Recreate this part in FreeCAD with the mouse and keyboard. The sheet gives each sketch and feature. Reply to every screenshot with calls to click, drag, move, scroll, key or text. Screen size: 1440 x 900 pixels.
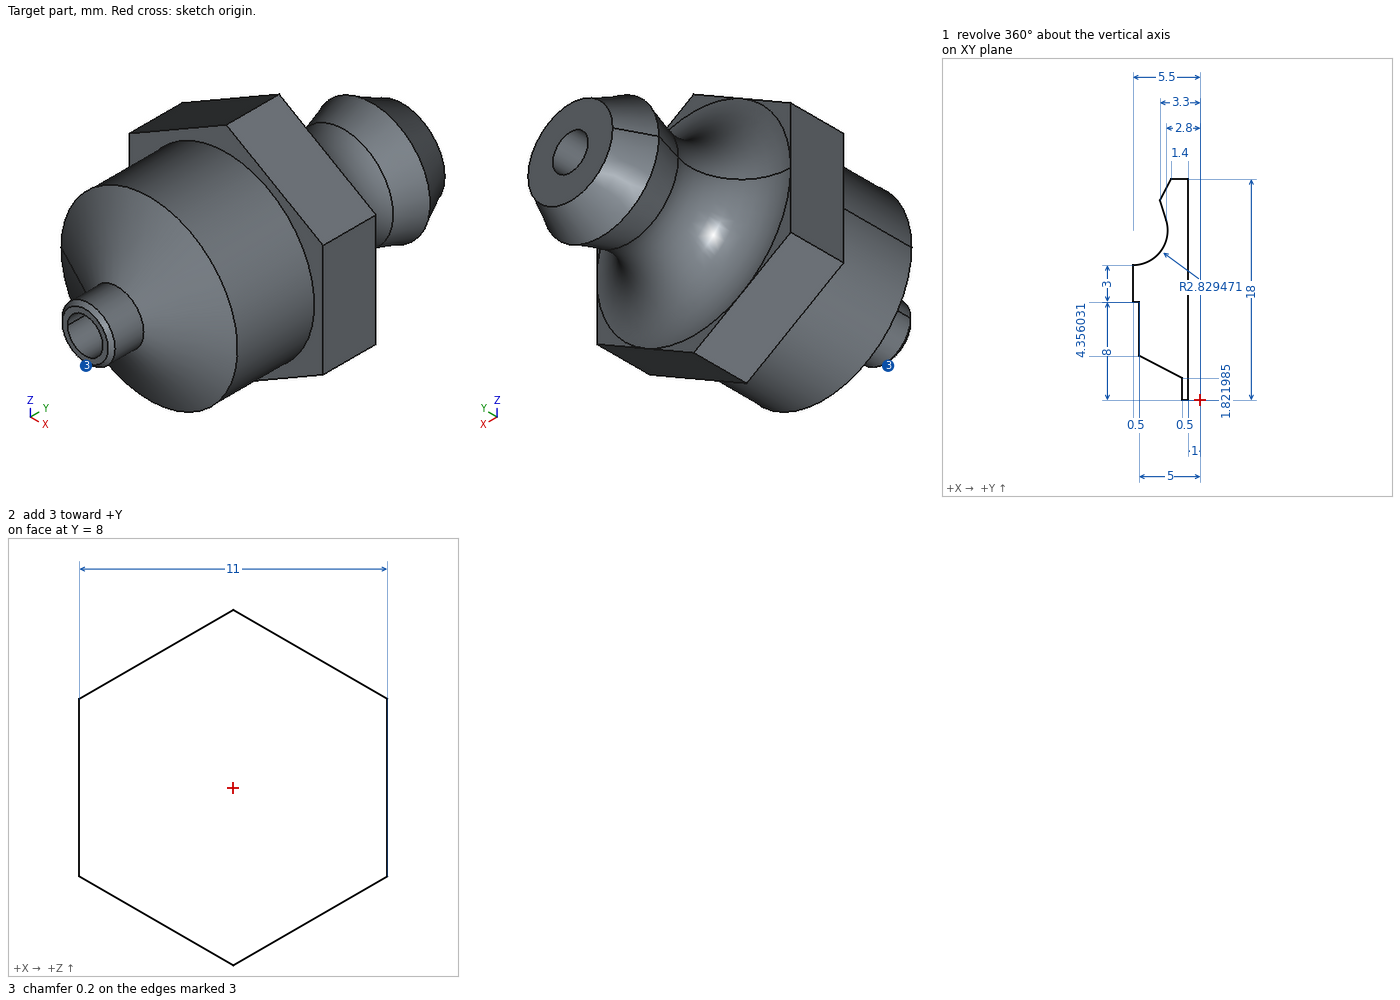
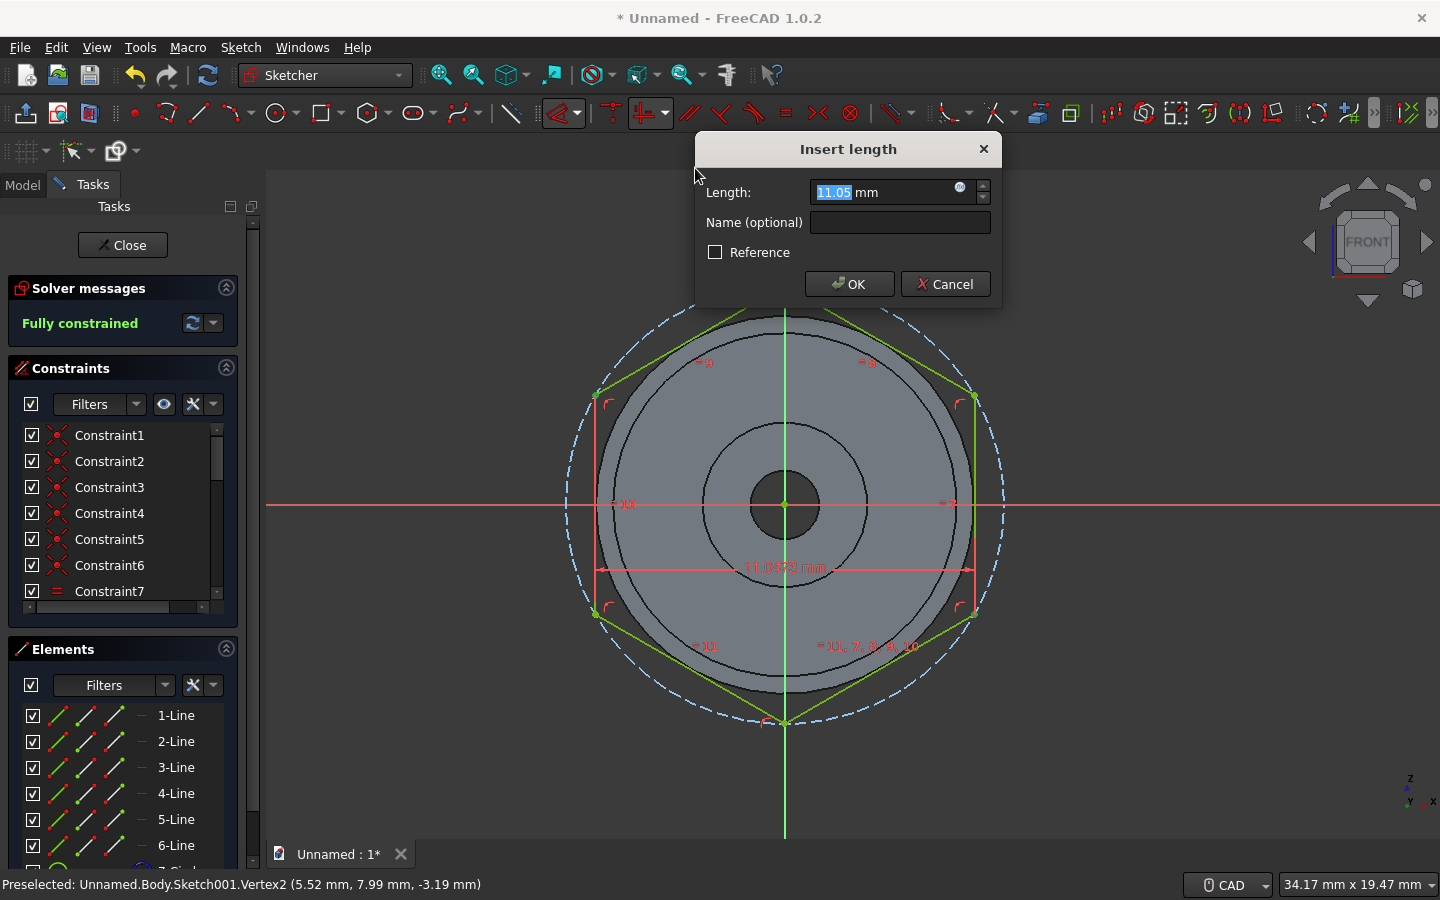
text(11)
key(Return)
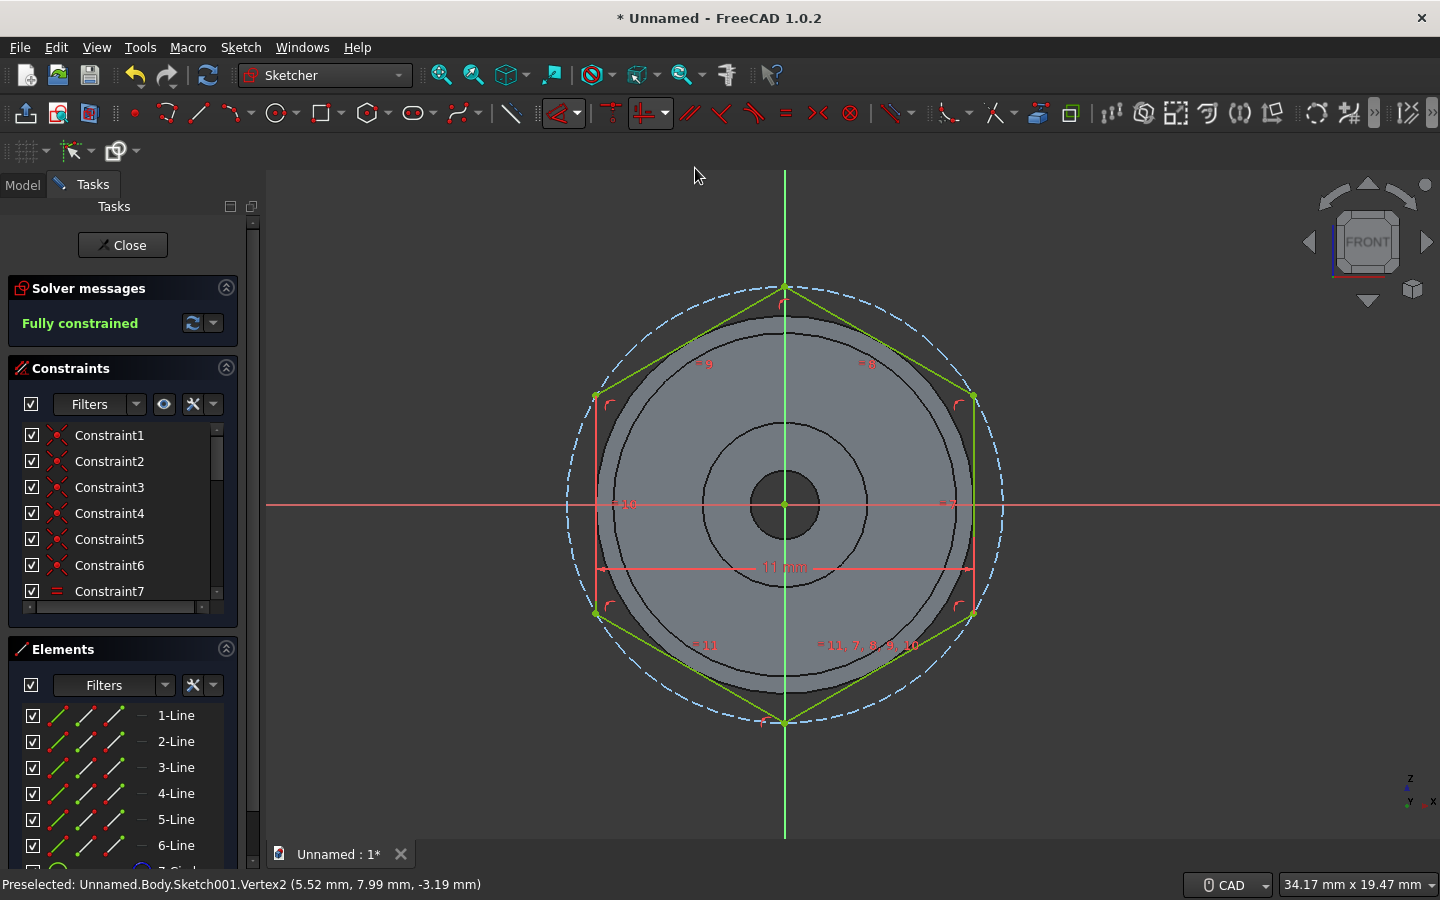
click(123, 245)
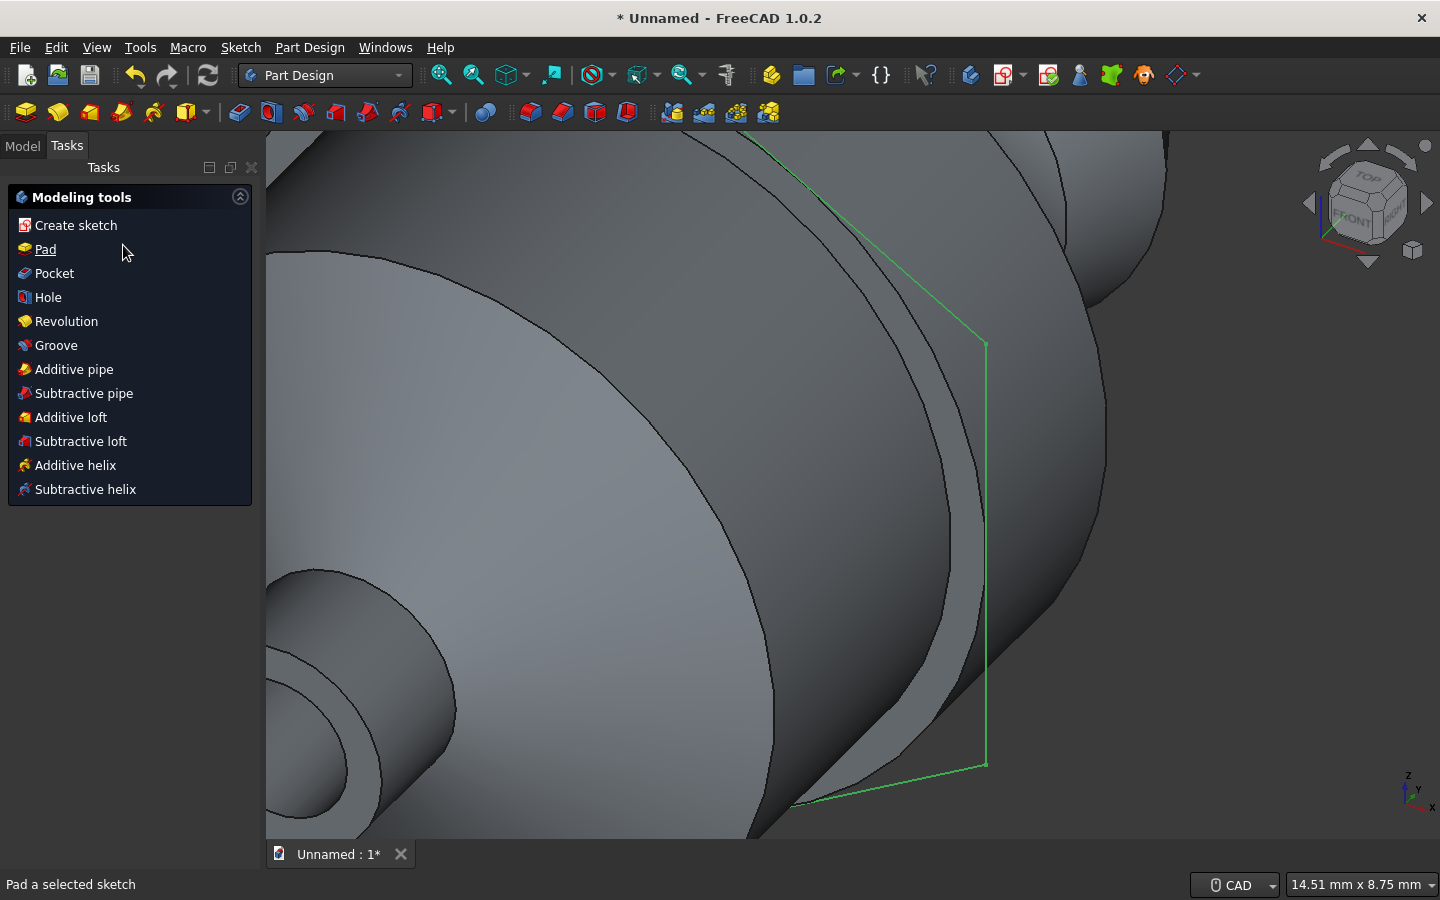
click(26, 112)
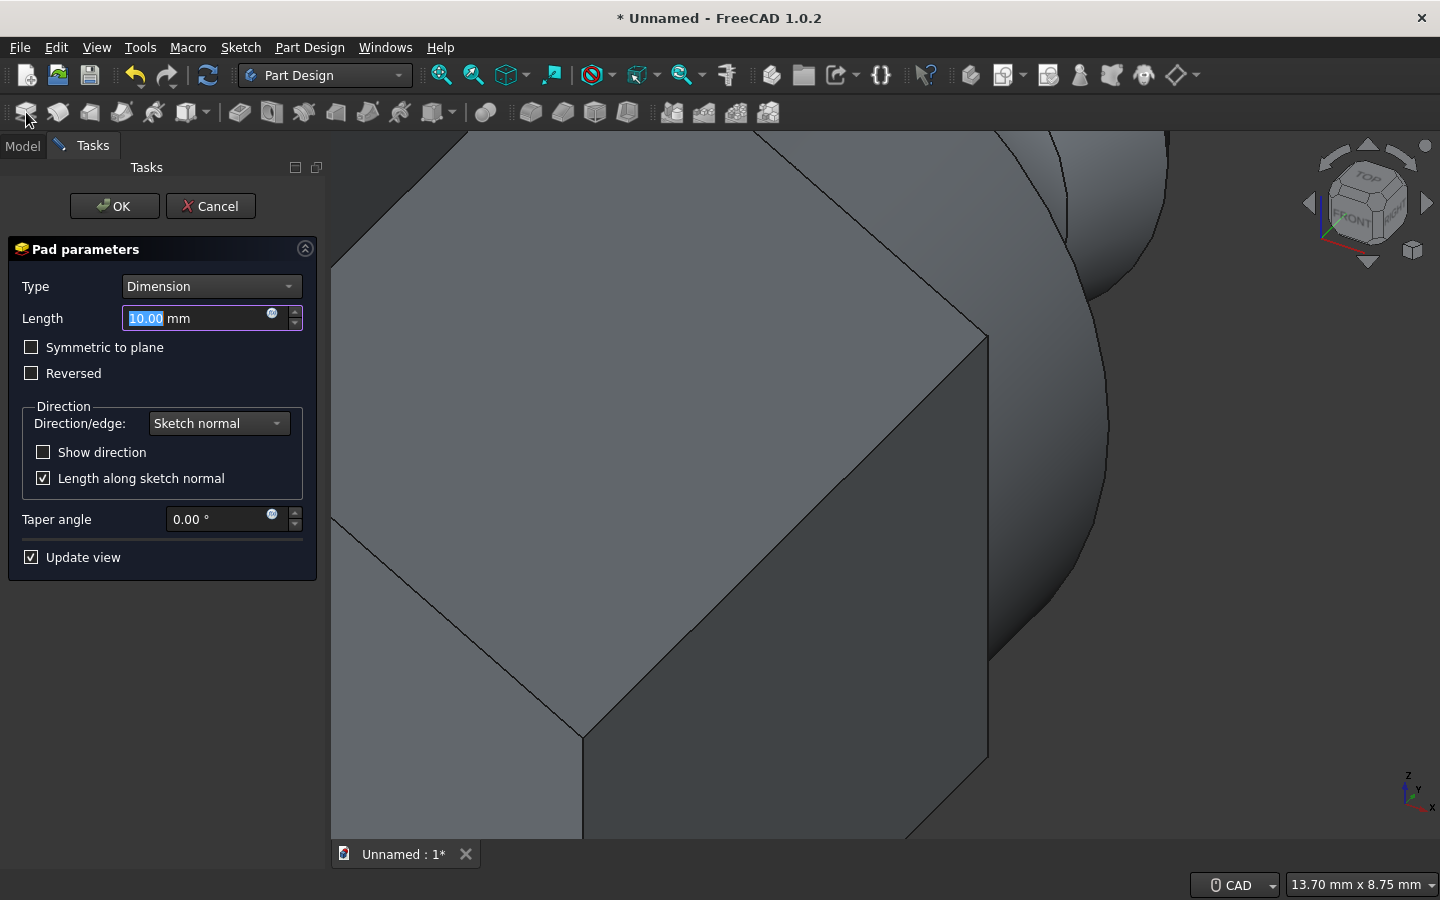
text(3)
key(Tab)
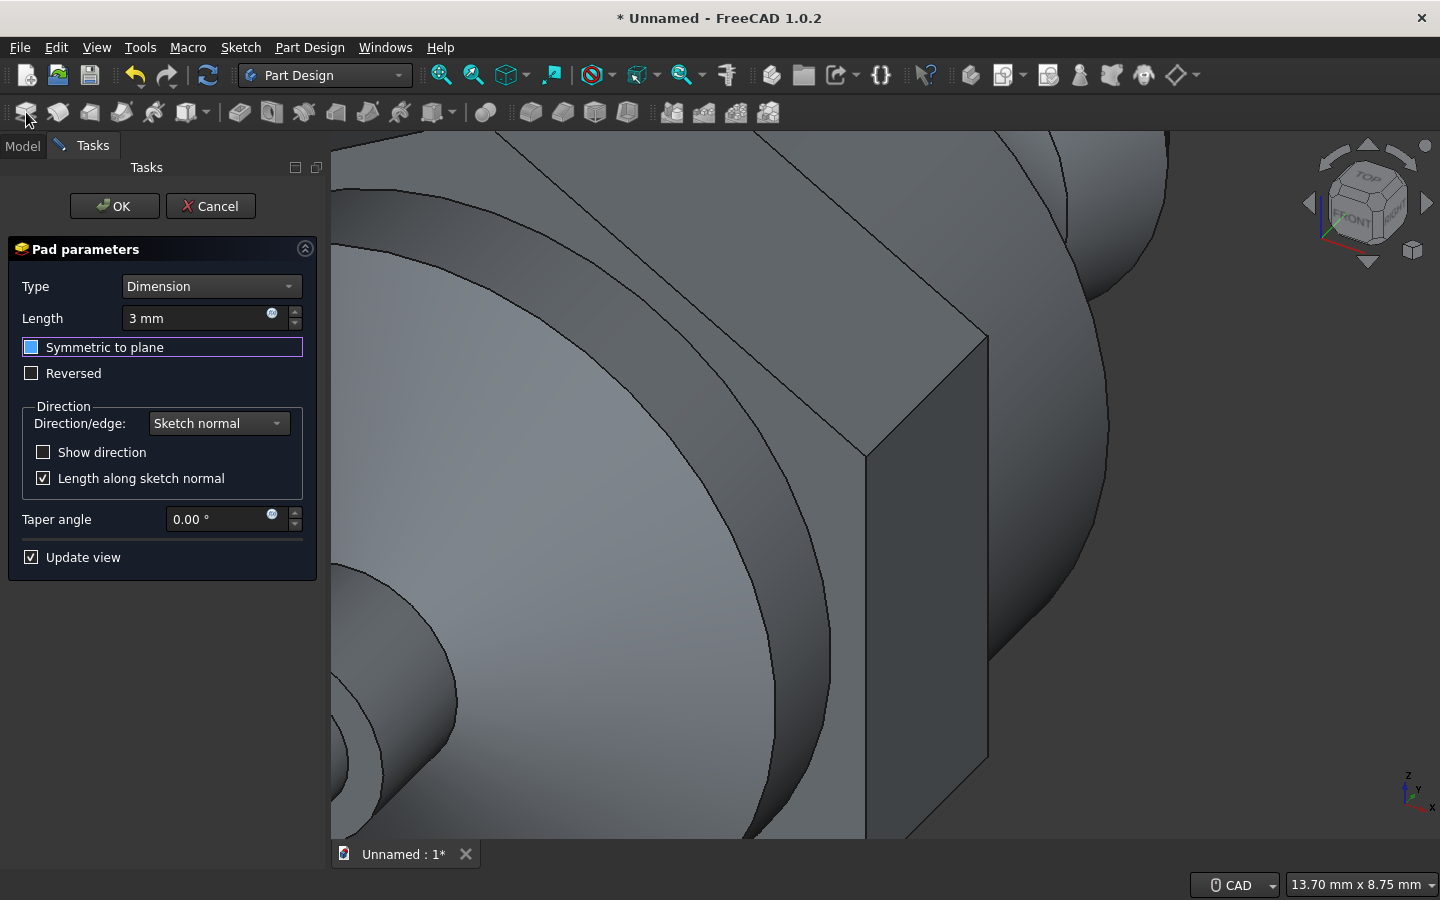
click(30, 373)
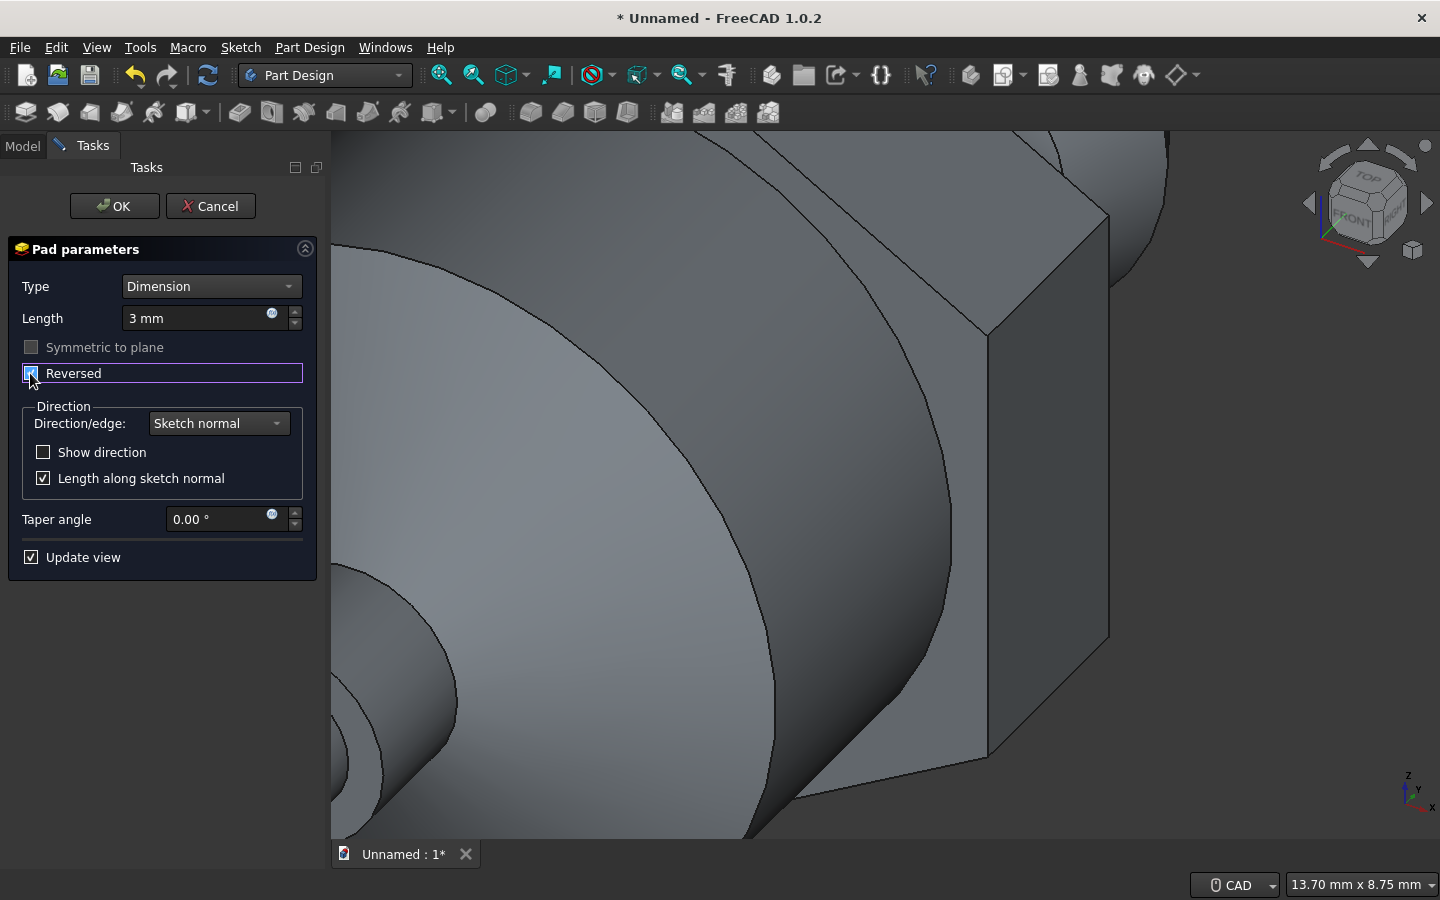
click(115, 206)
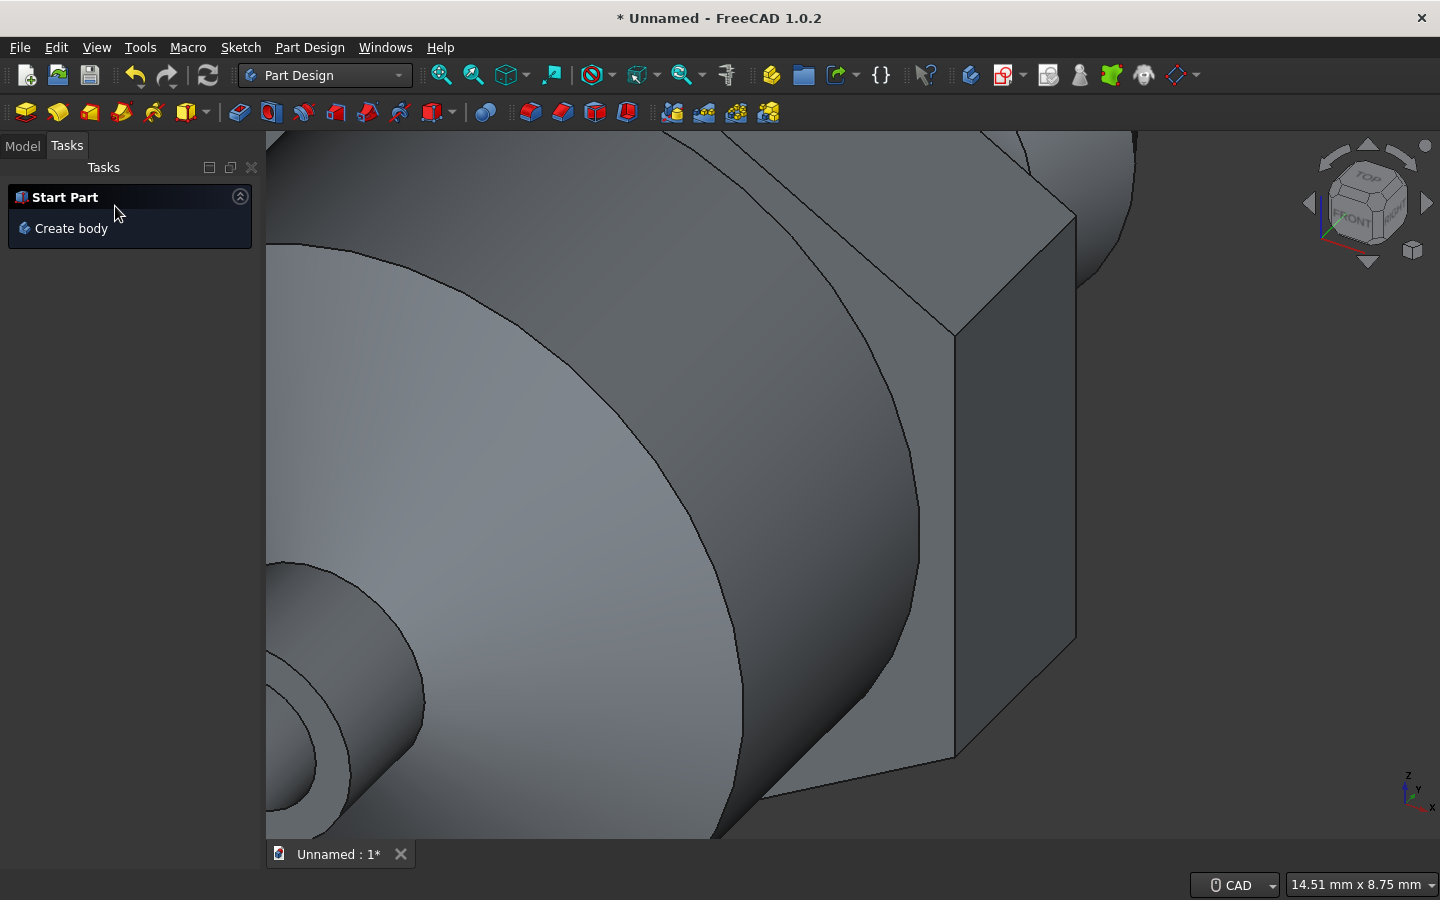
click(442, 76)